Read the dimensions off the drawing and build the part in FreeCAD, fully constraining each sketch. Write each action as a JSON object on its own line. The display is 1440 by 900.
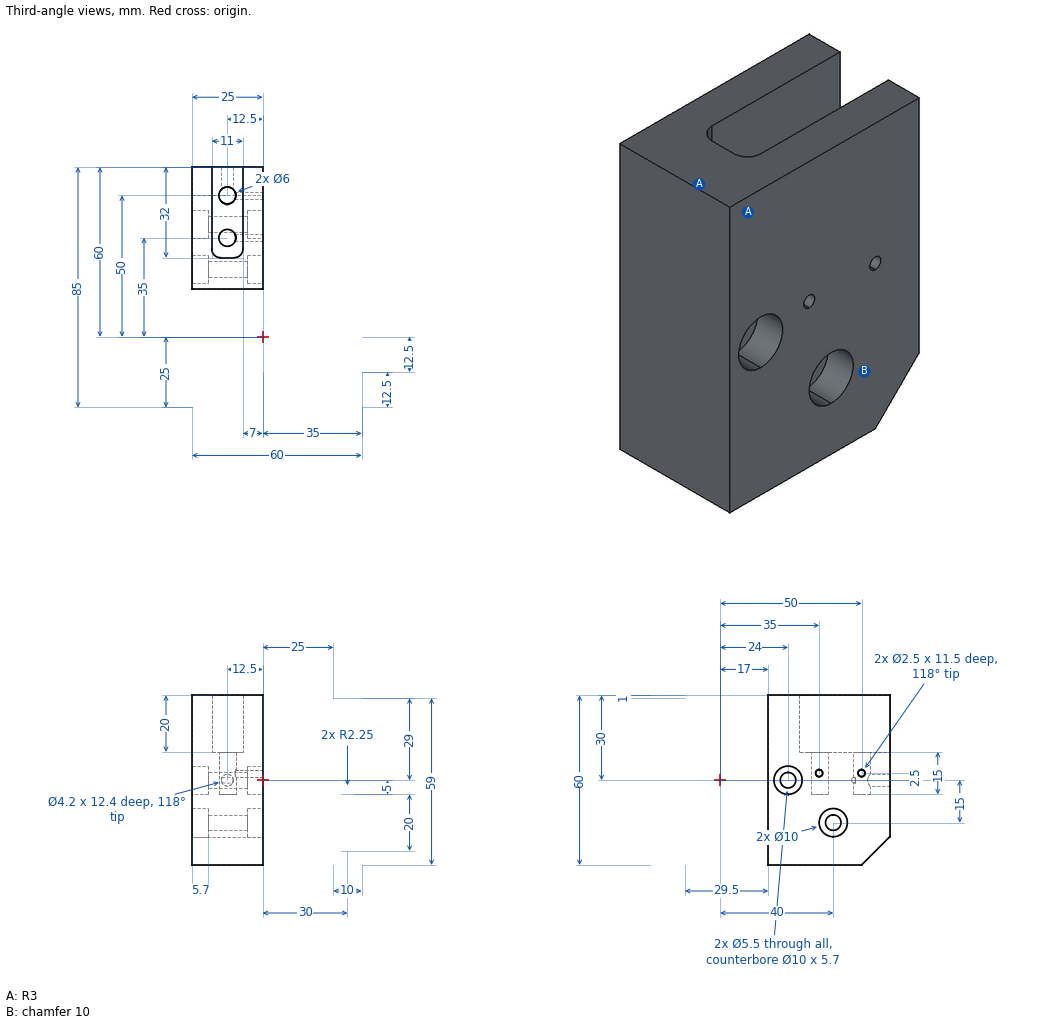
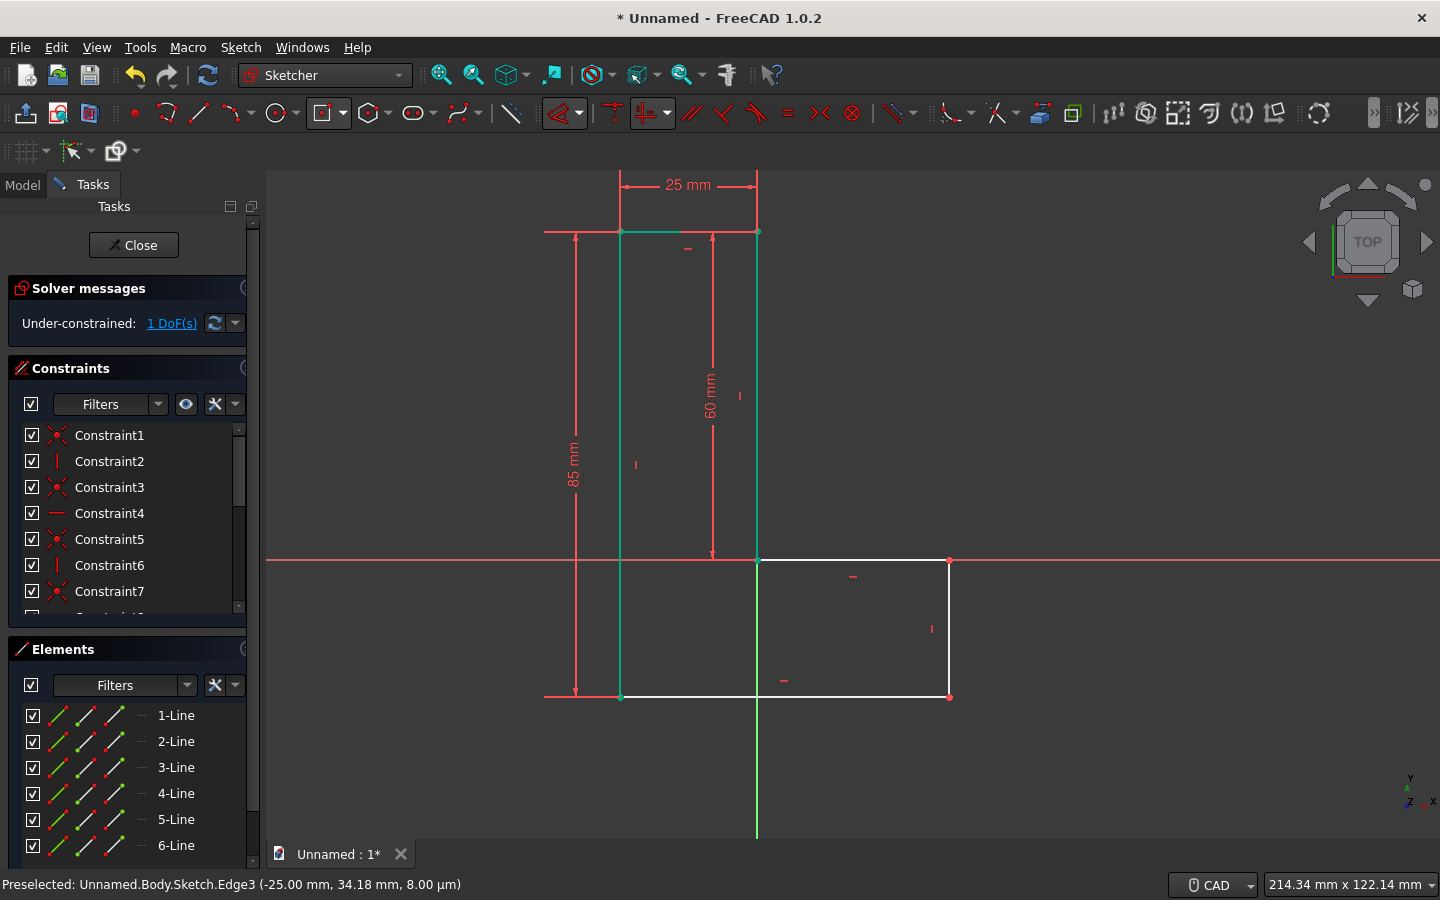
{"action": "left_click", "coordinate": [719, 697]}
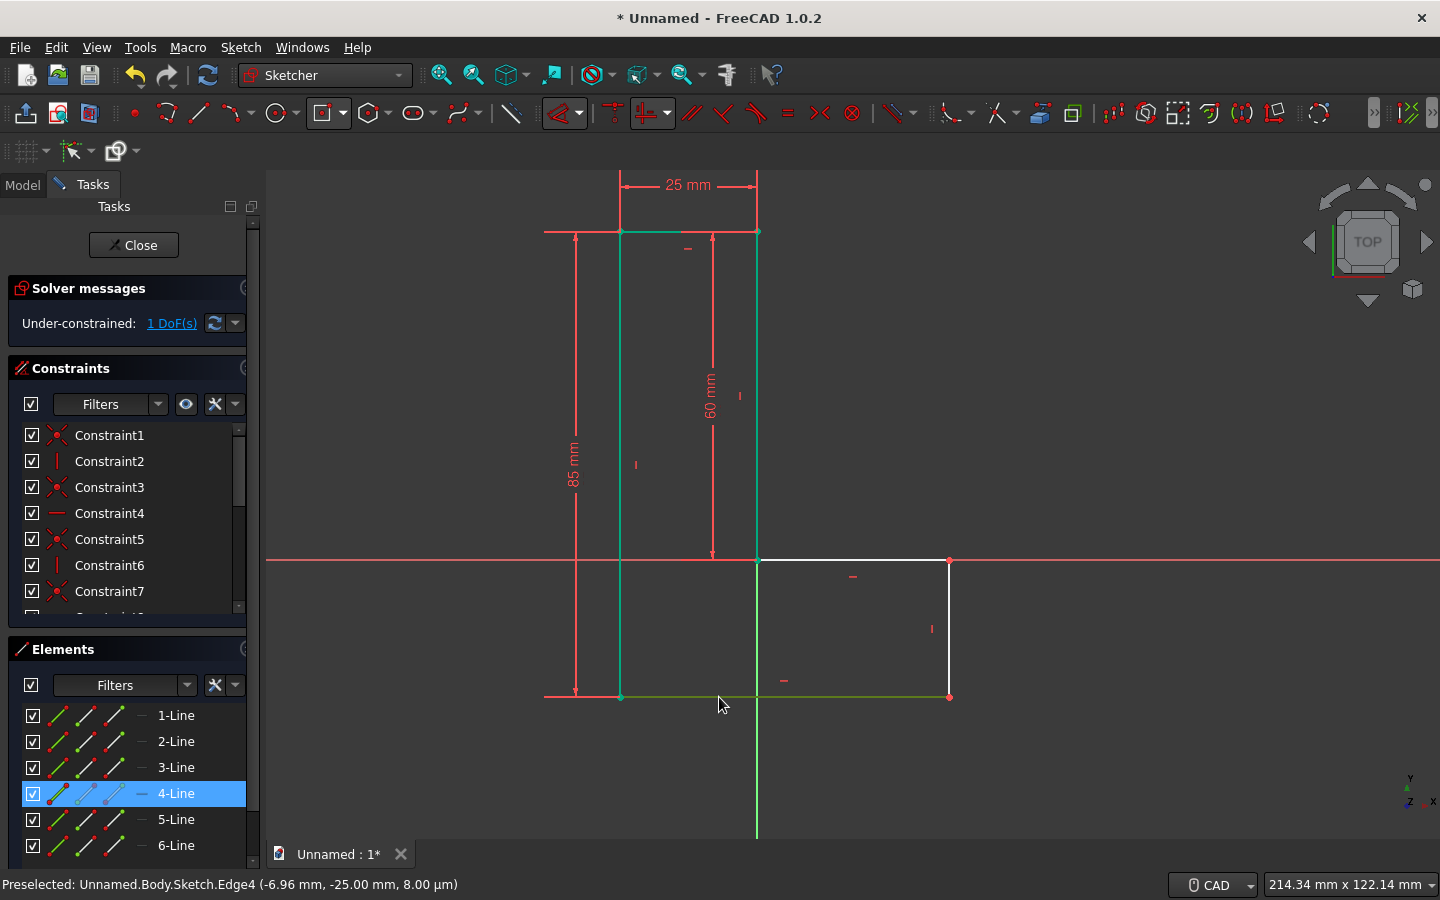
{"action": "key", "text": "l"}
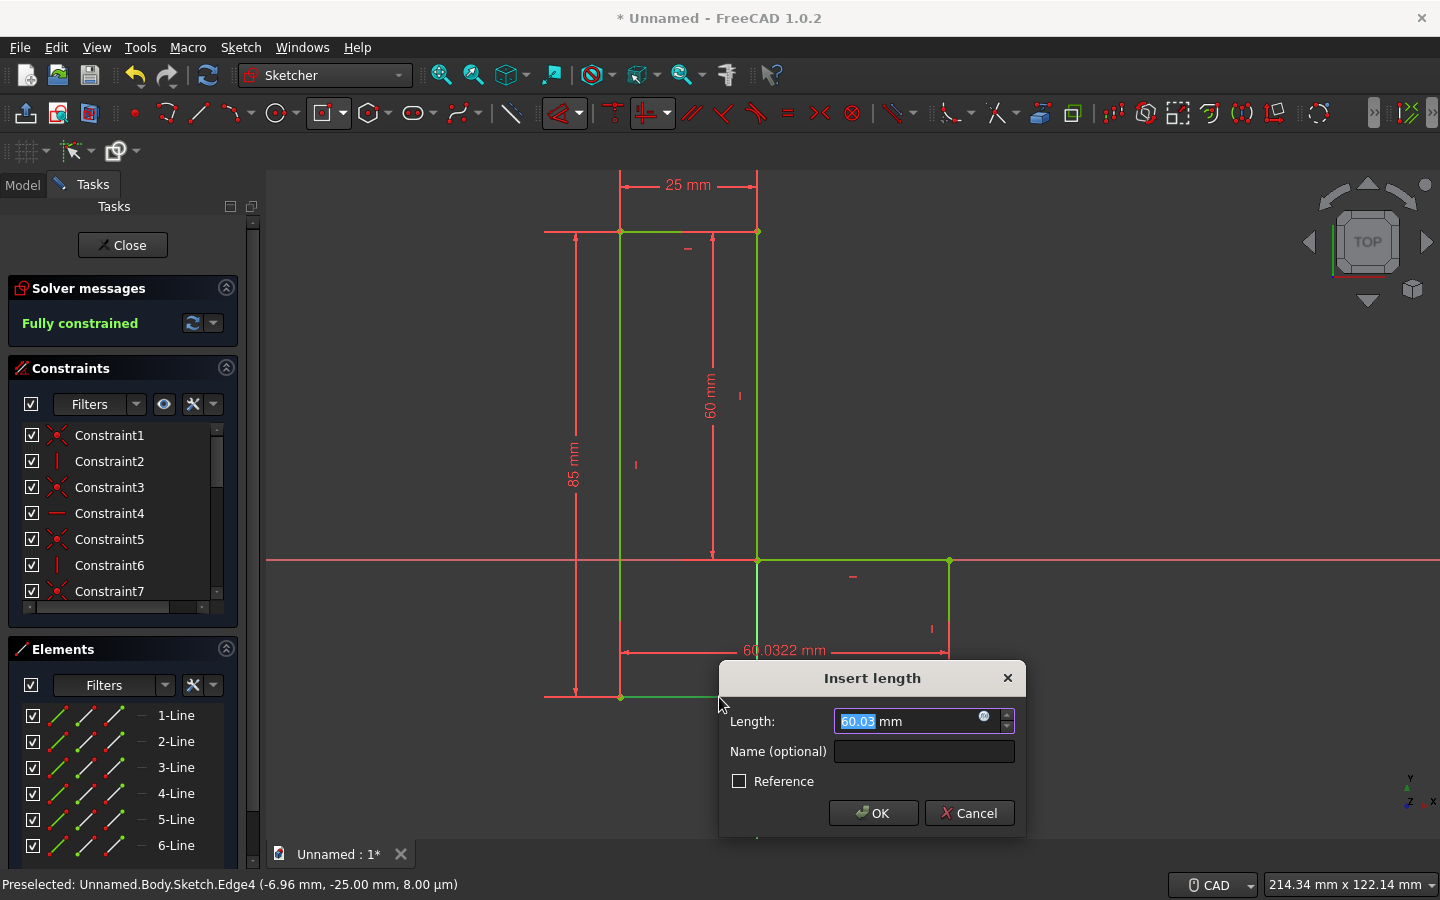
{"action": "type", "text": "60"}
{"action": "key", "text": "Return"}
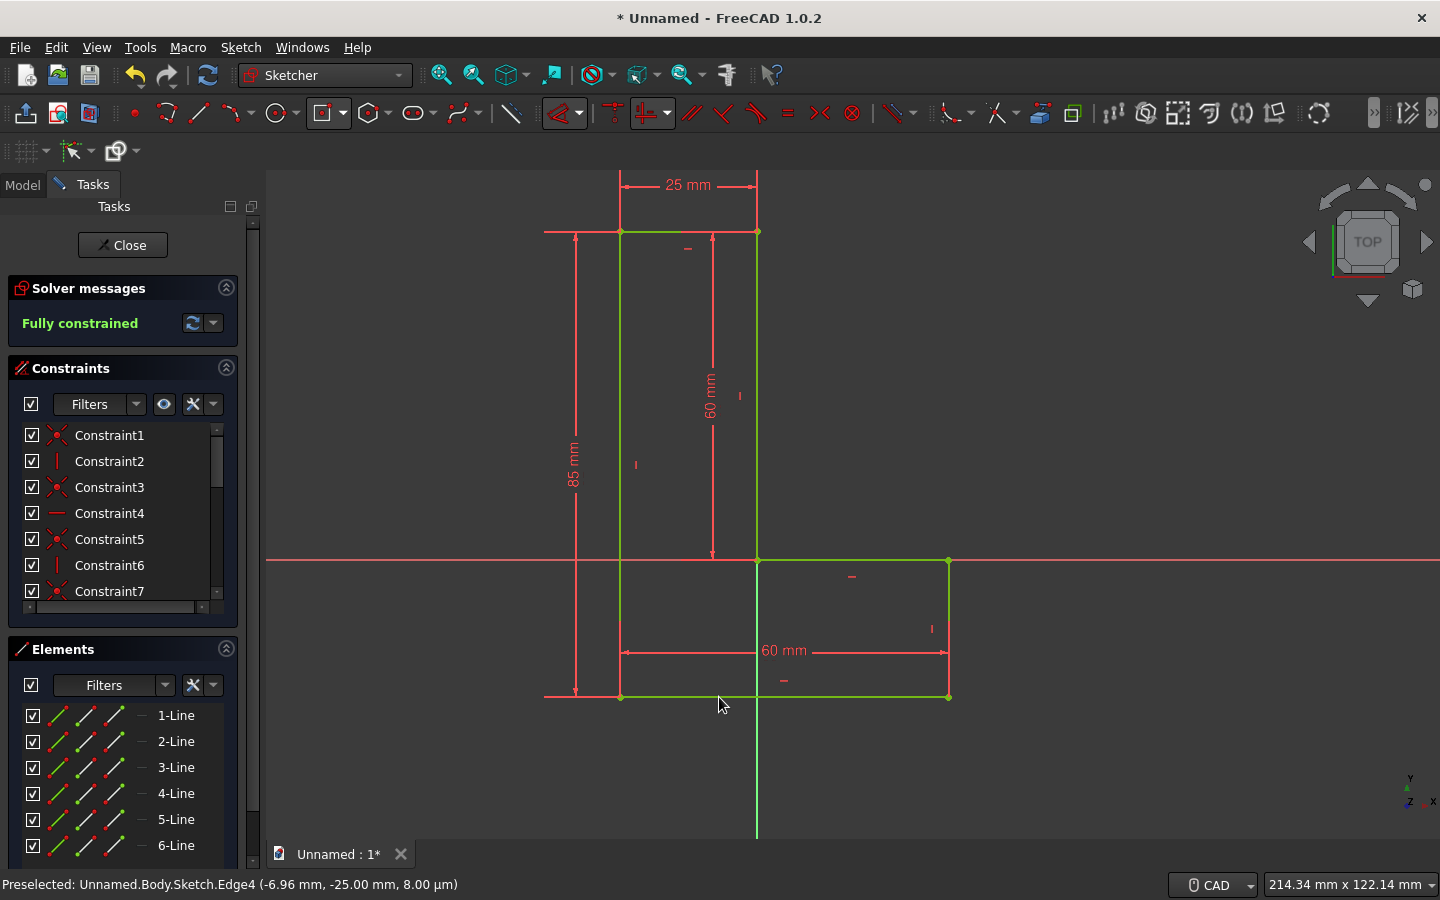
{"action": "left_click", "coordinate": [123, 245]}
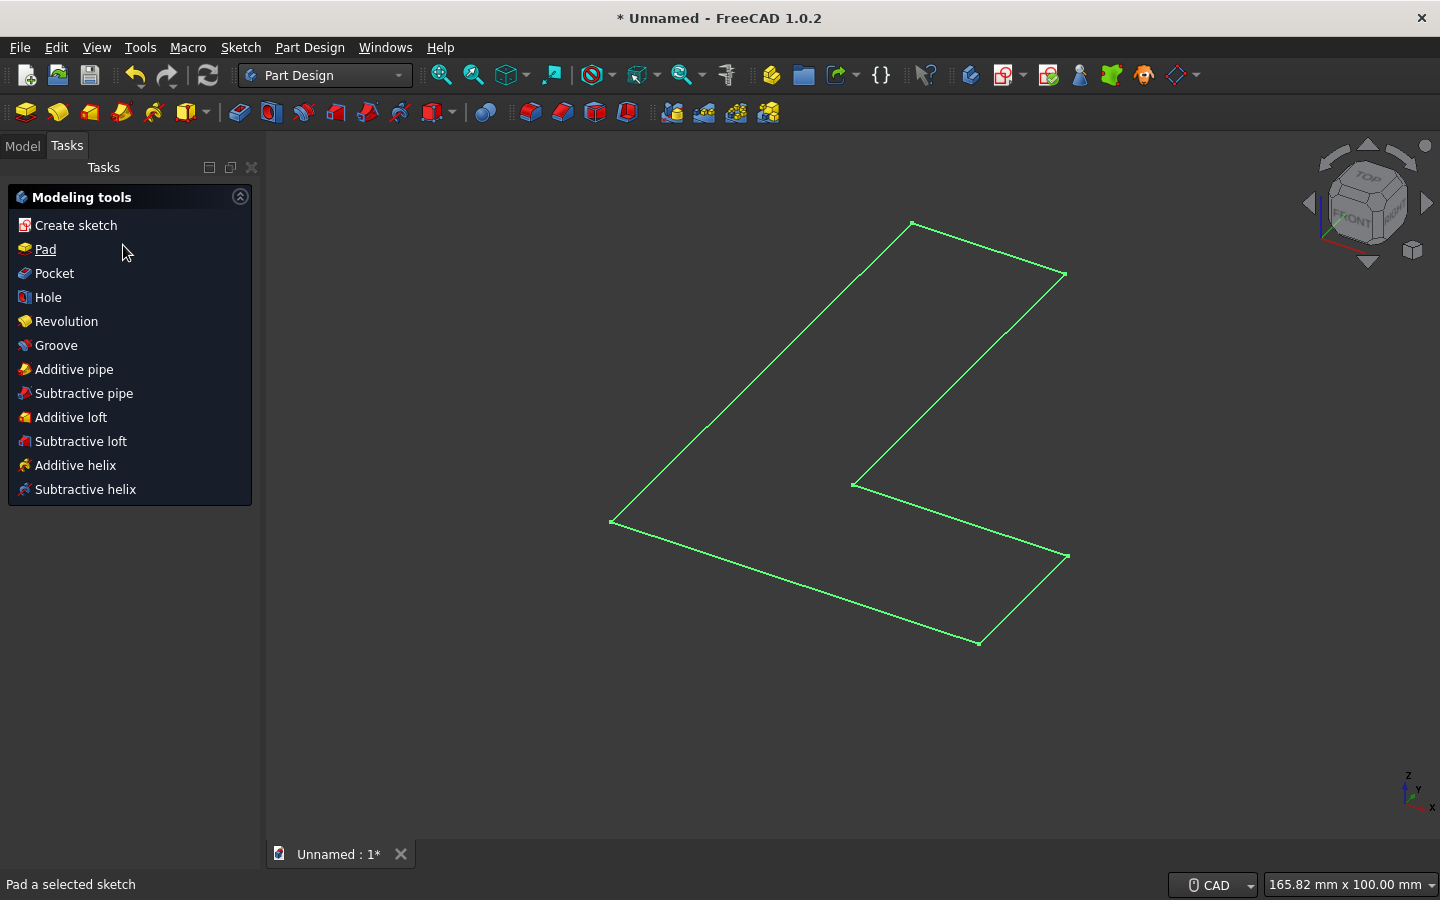
{"action": "left_click", "coordinate": [26, 112]}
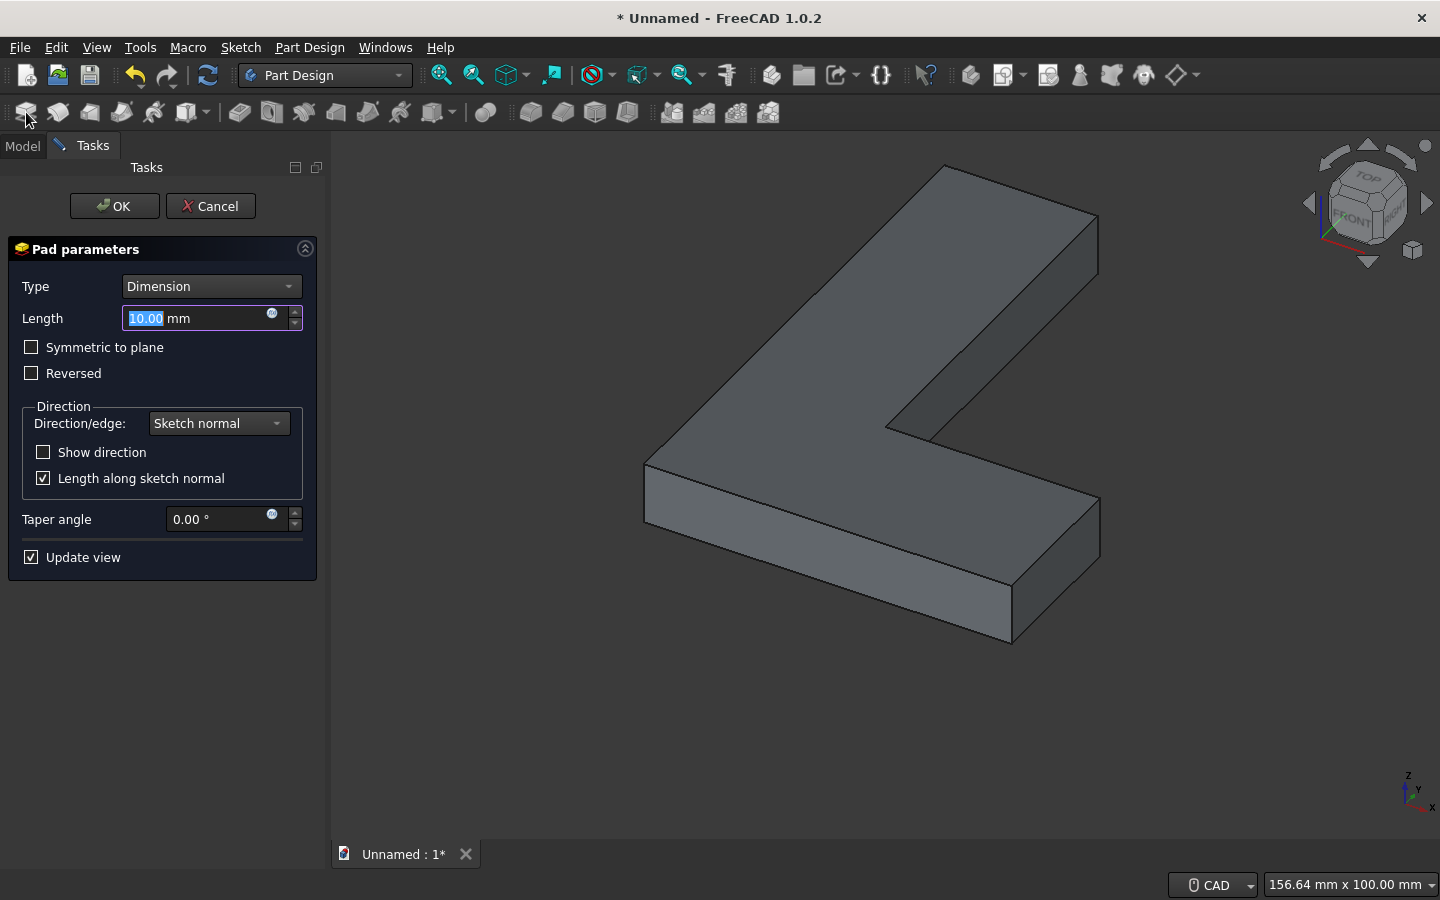
{"action": "type", "text": "60"}
{"action": "key", "text": "Tab"}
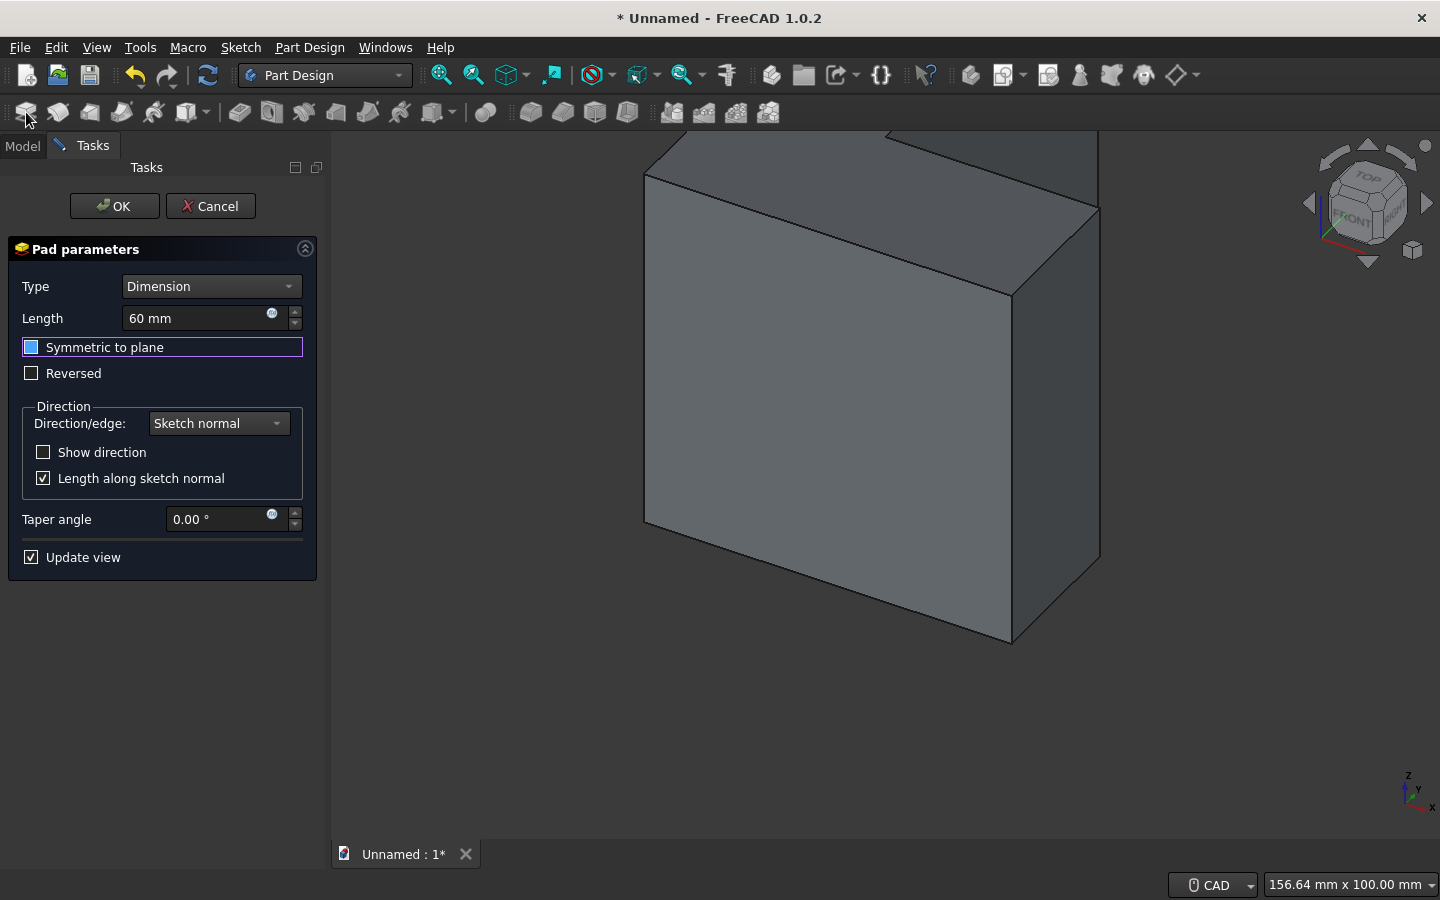
{"action": "left_click", "coordinate": [30, 347]}